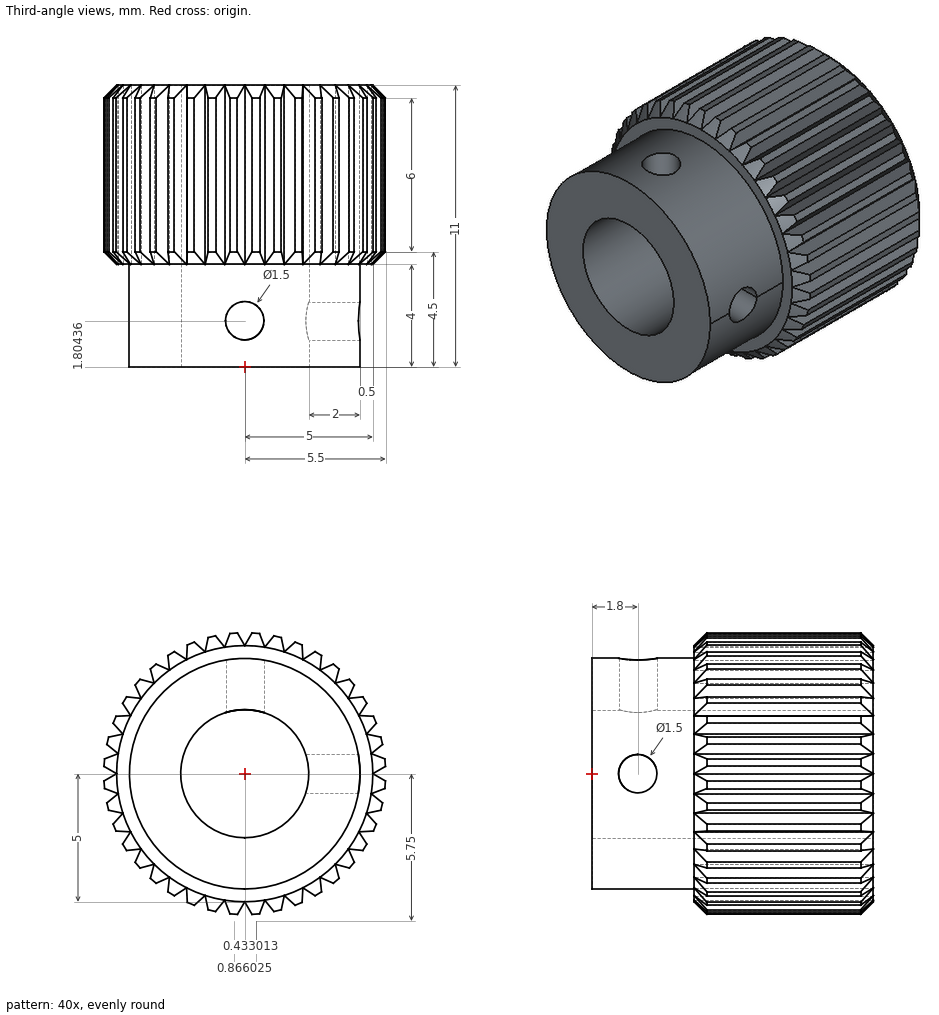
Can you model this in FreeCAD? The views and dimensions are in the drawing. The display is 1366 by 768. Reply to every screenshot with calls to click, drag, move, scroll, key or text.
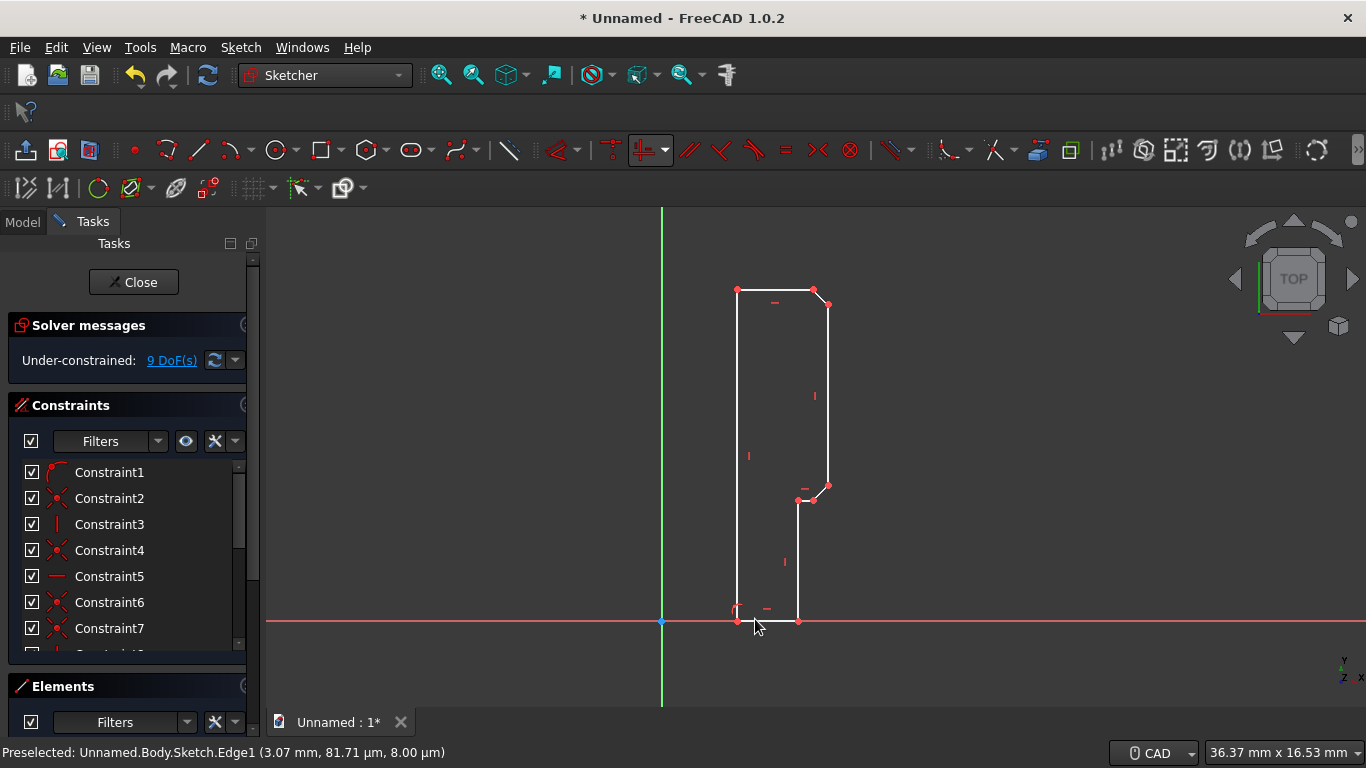
click(755, 621)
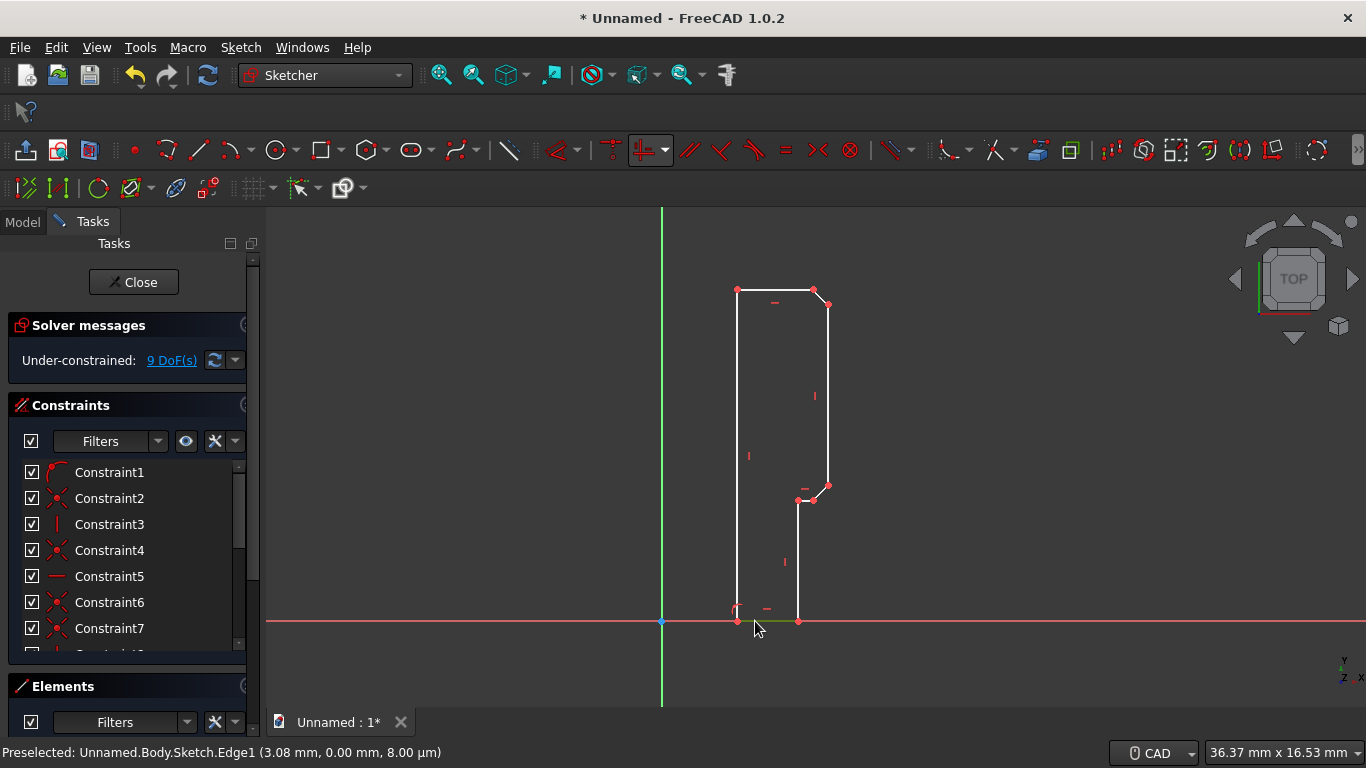
key(l)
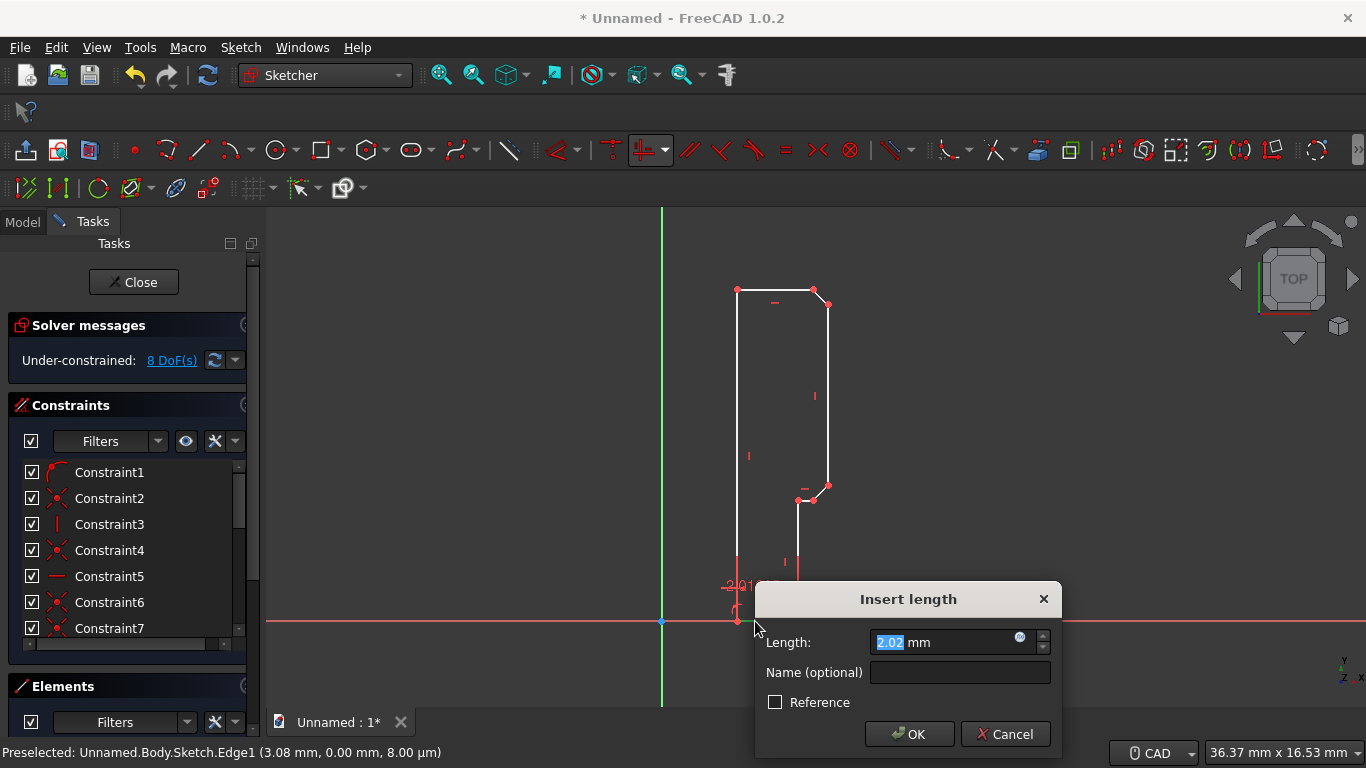
text(2)
key(Return)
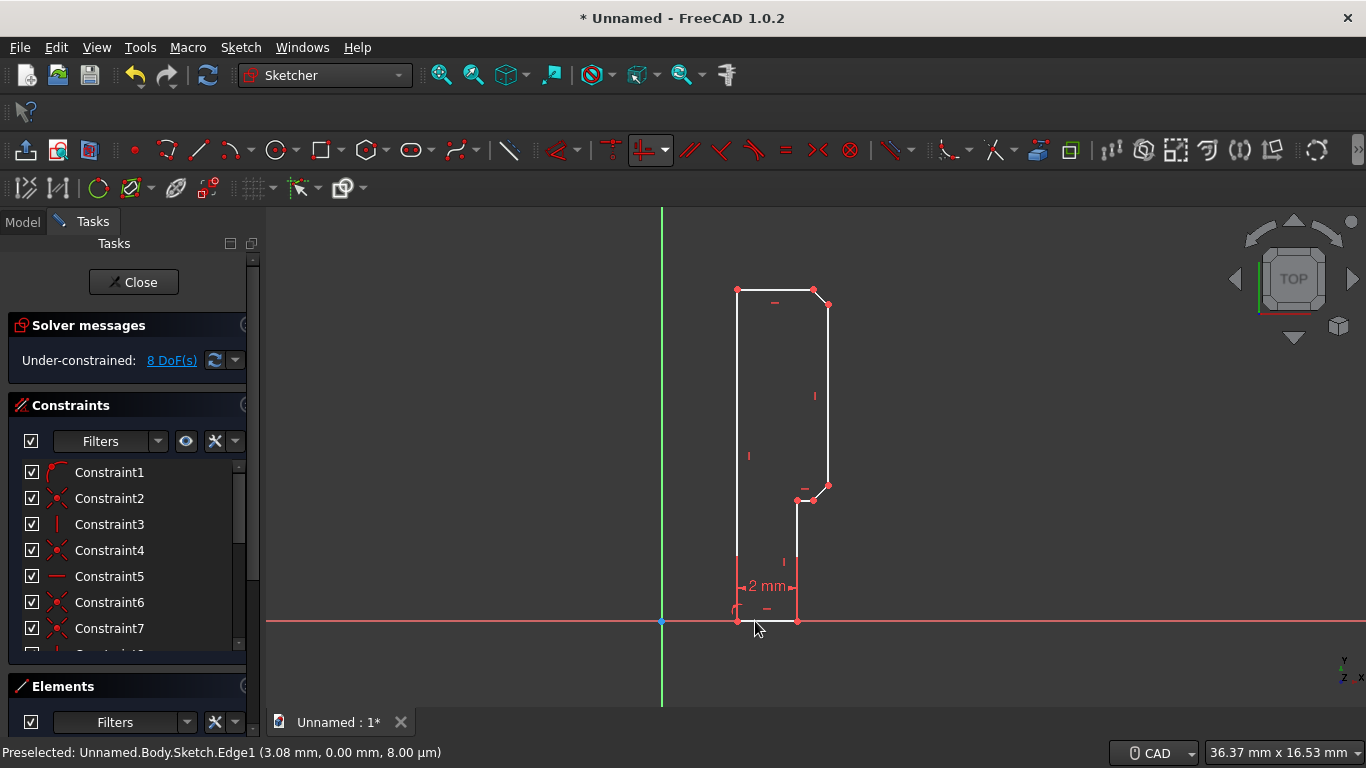
click(797, 585)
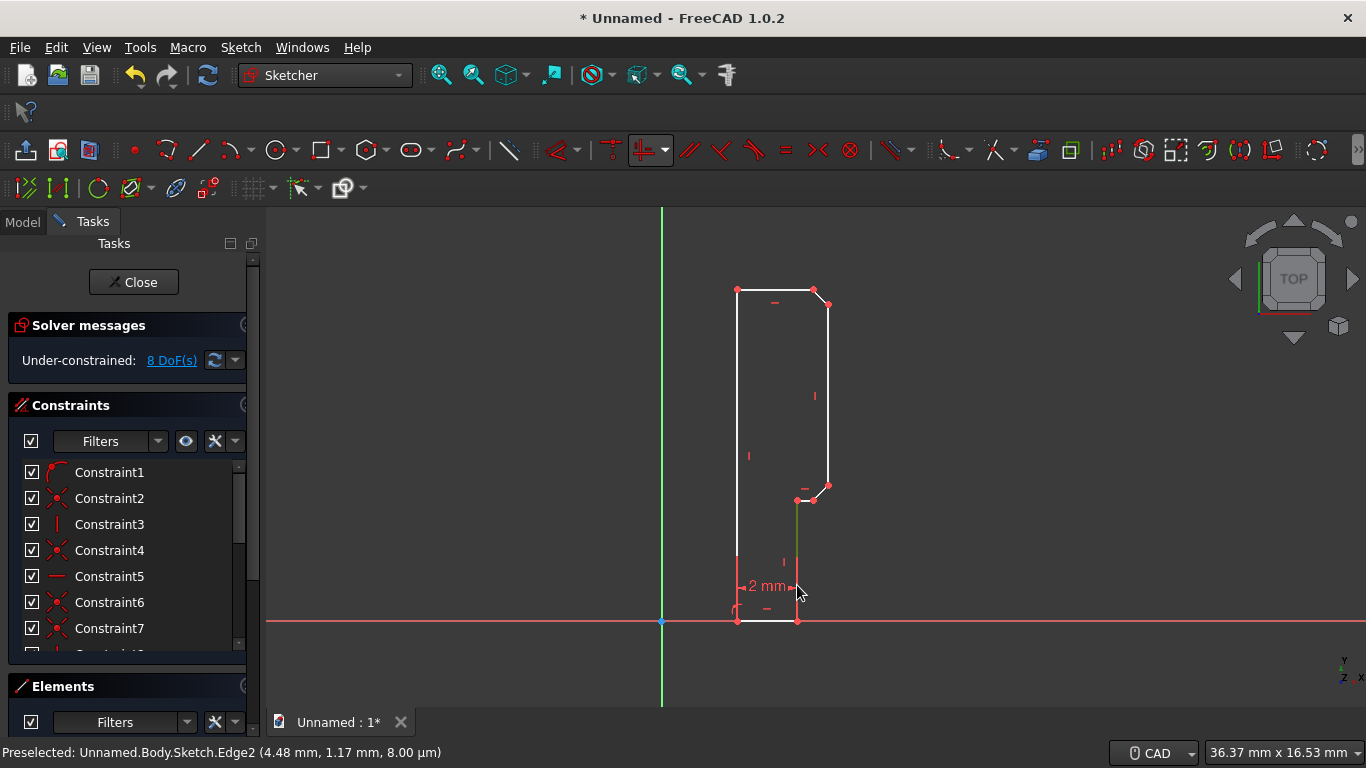
key(i)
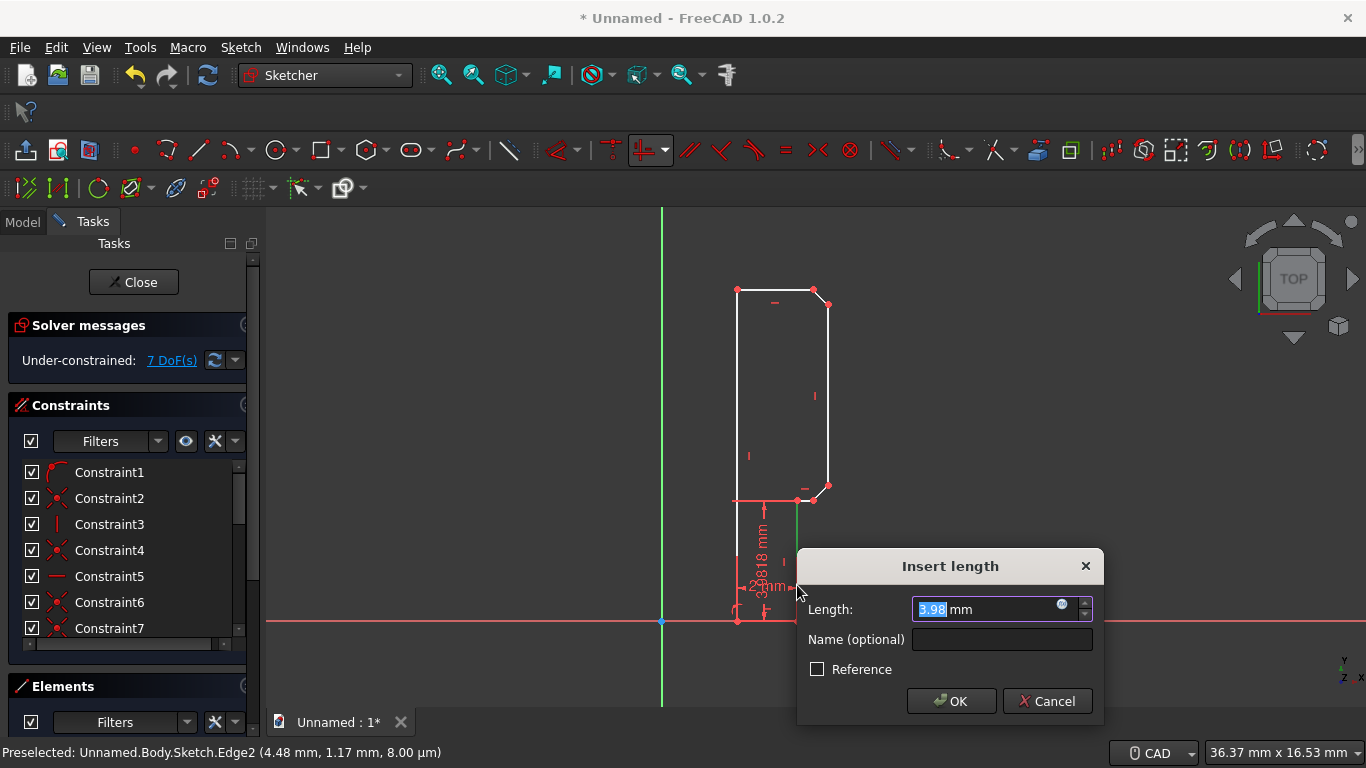
text(4)
key(Return)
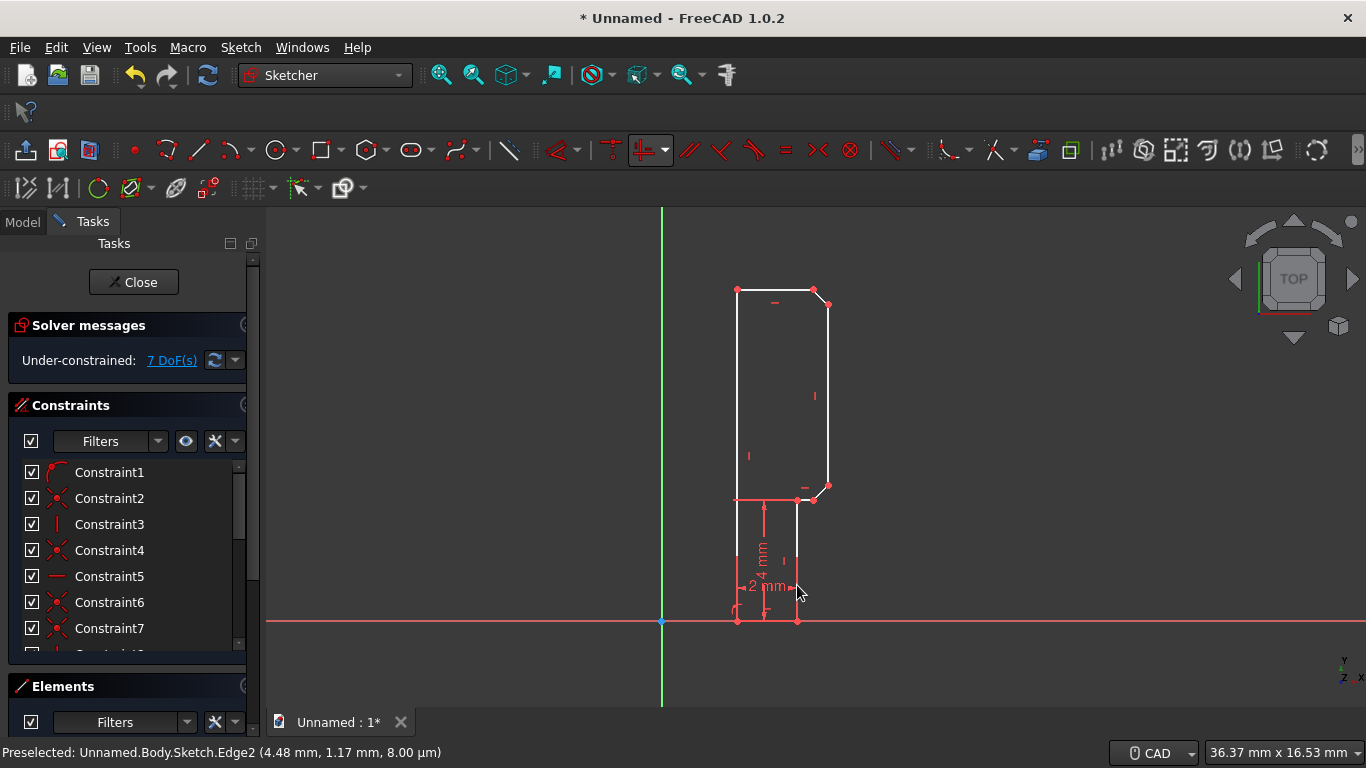
click(828, 432)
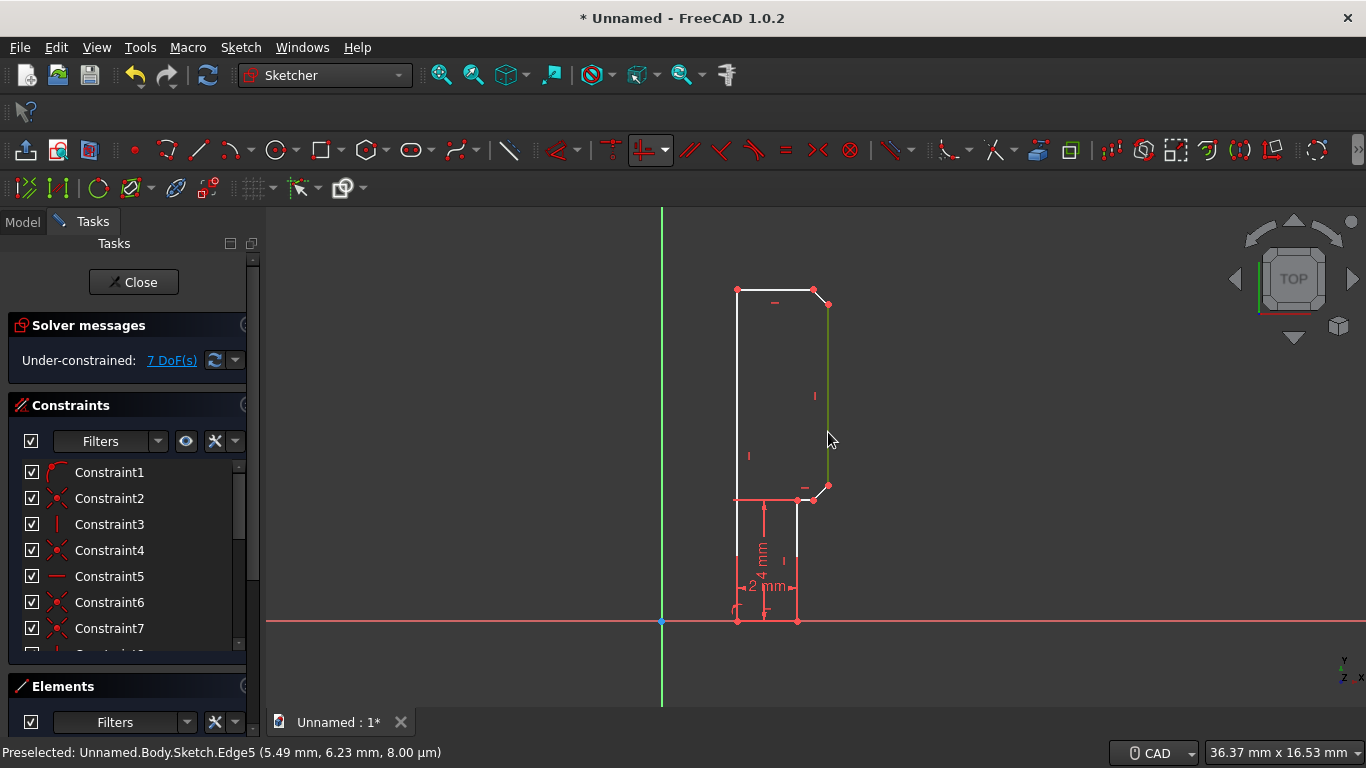
key(i)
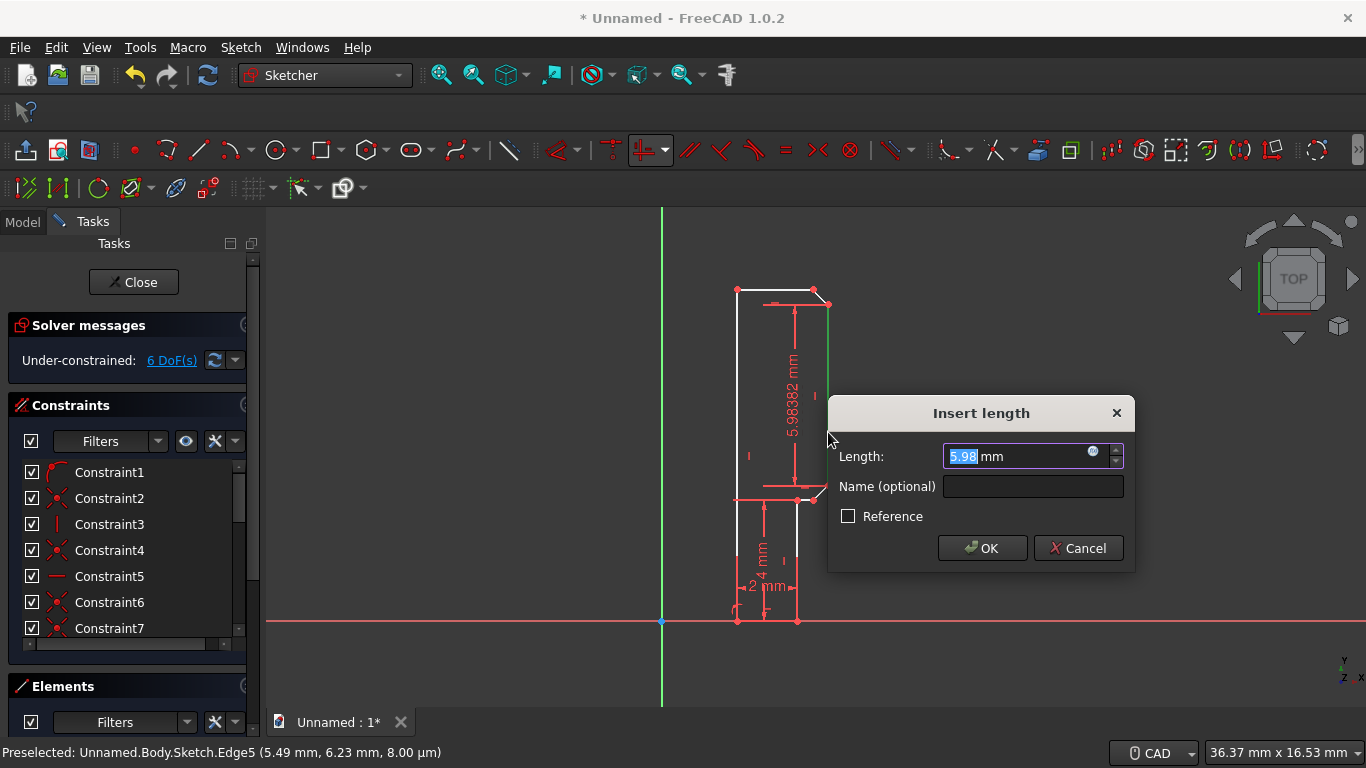
text(6)
key(Return)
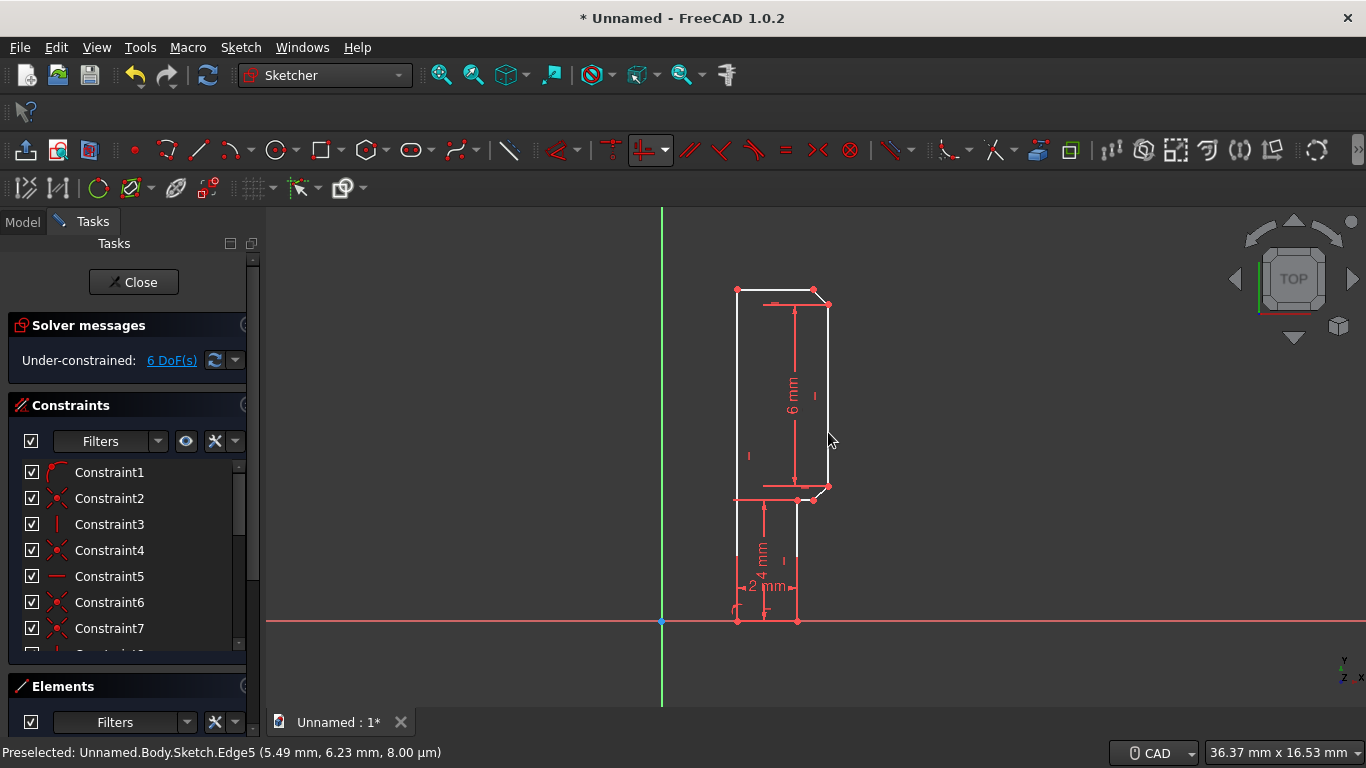
click(737, 389)